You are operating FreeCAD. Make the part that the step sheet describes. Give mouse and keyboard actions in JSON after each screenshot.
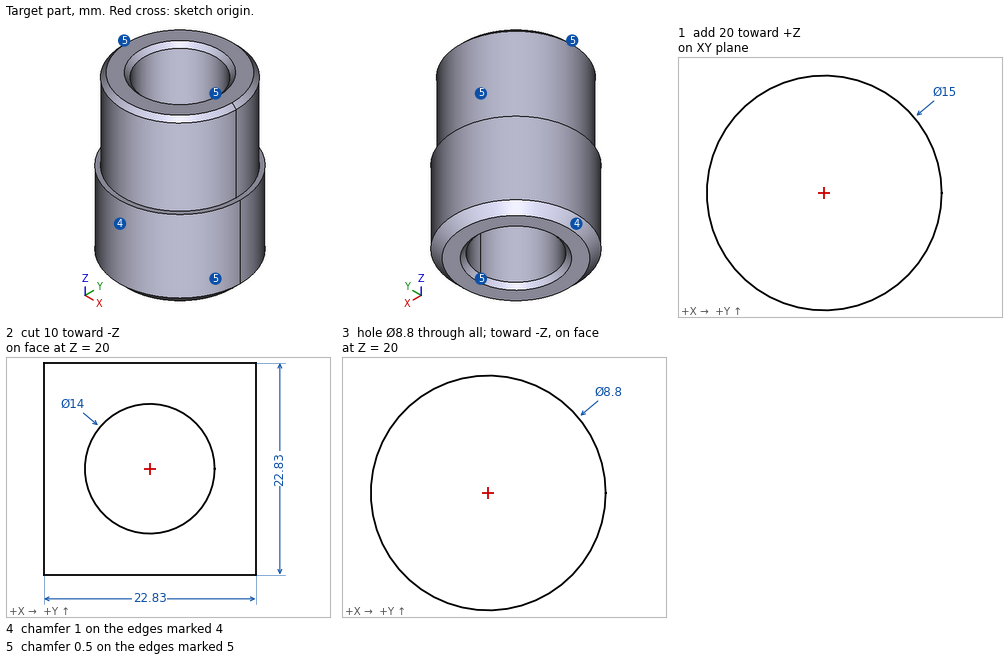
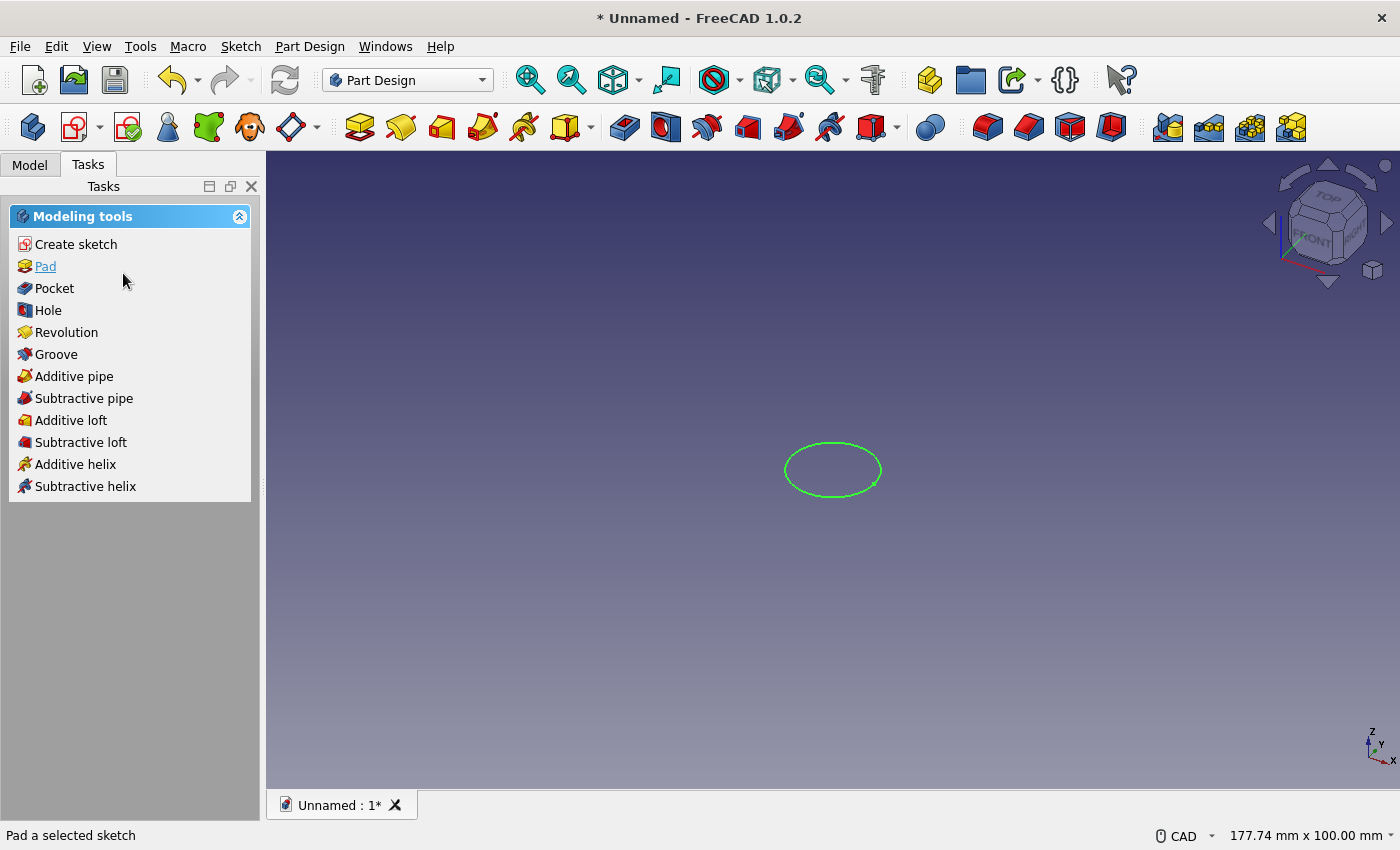
{"action": "left_click", "coordinate": [360, 128]}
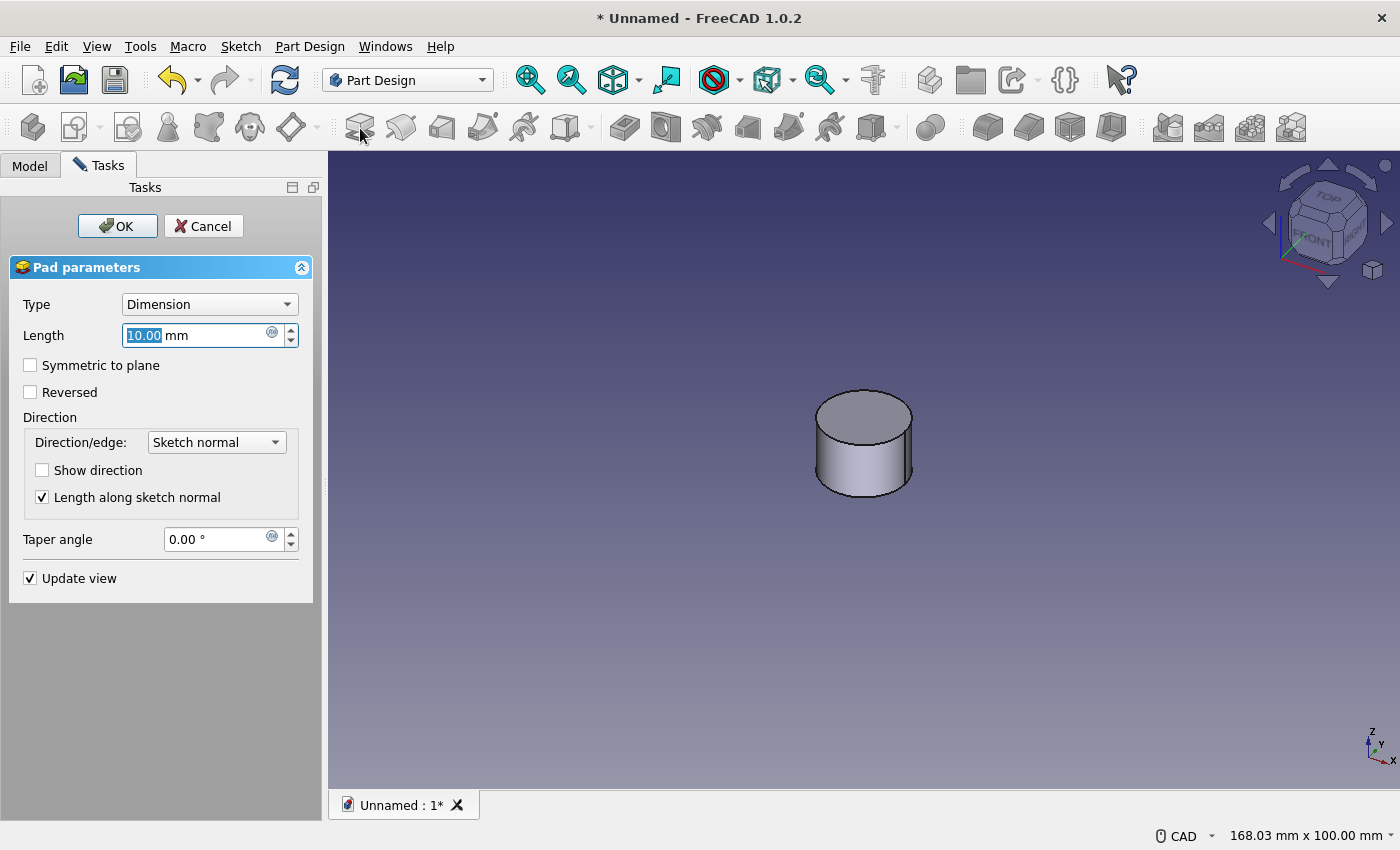
{"action": "type", "text": "20"}
{"action": "key", "text": "Tab"}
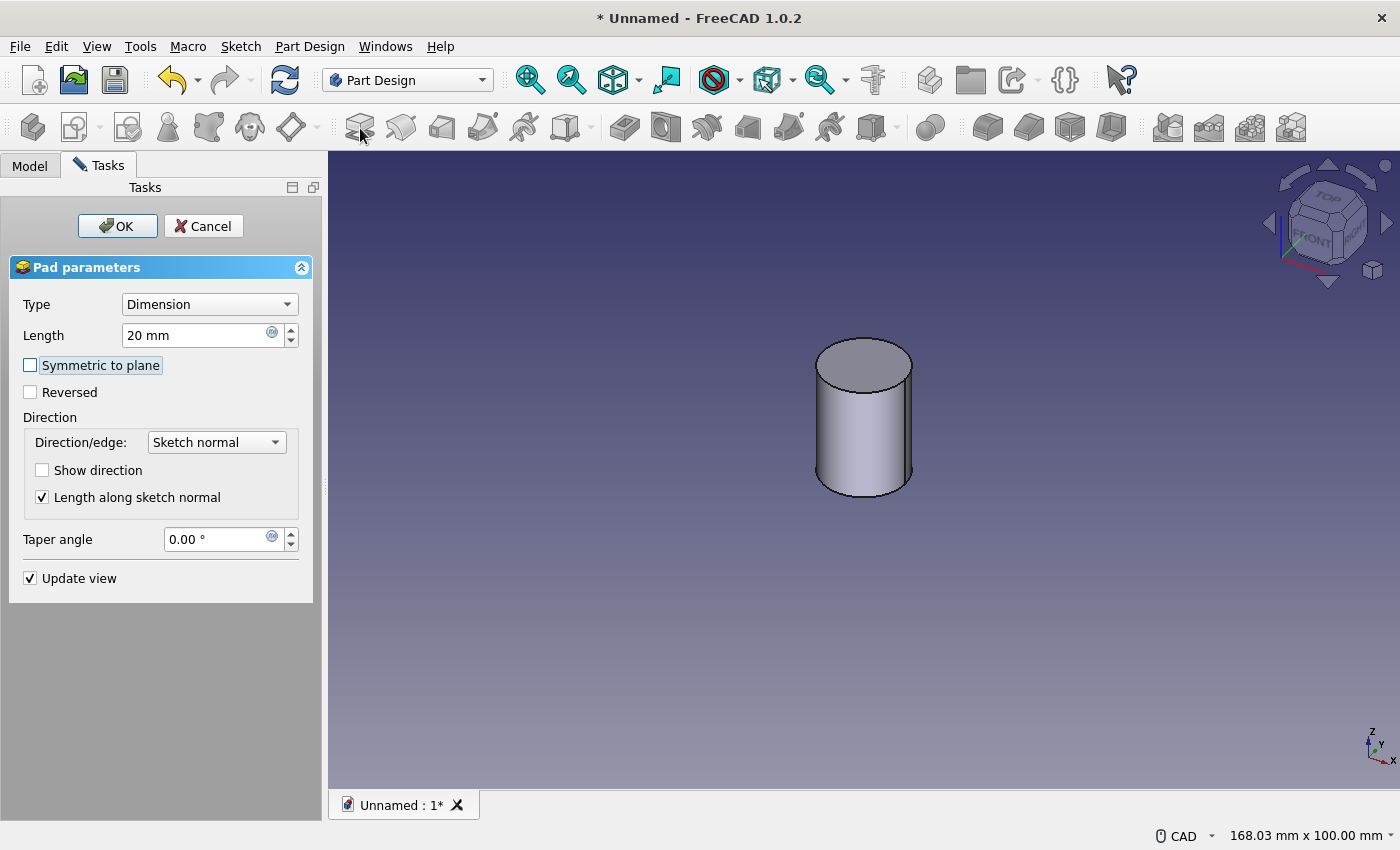
{"action": "left_click", "coordinate": [118, 226]}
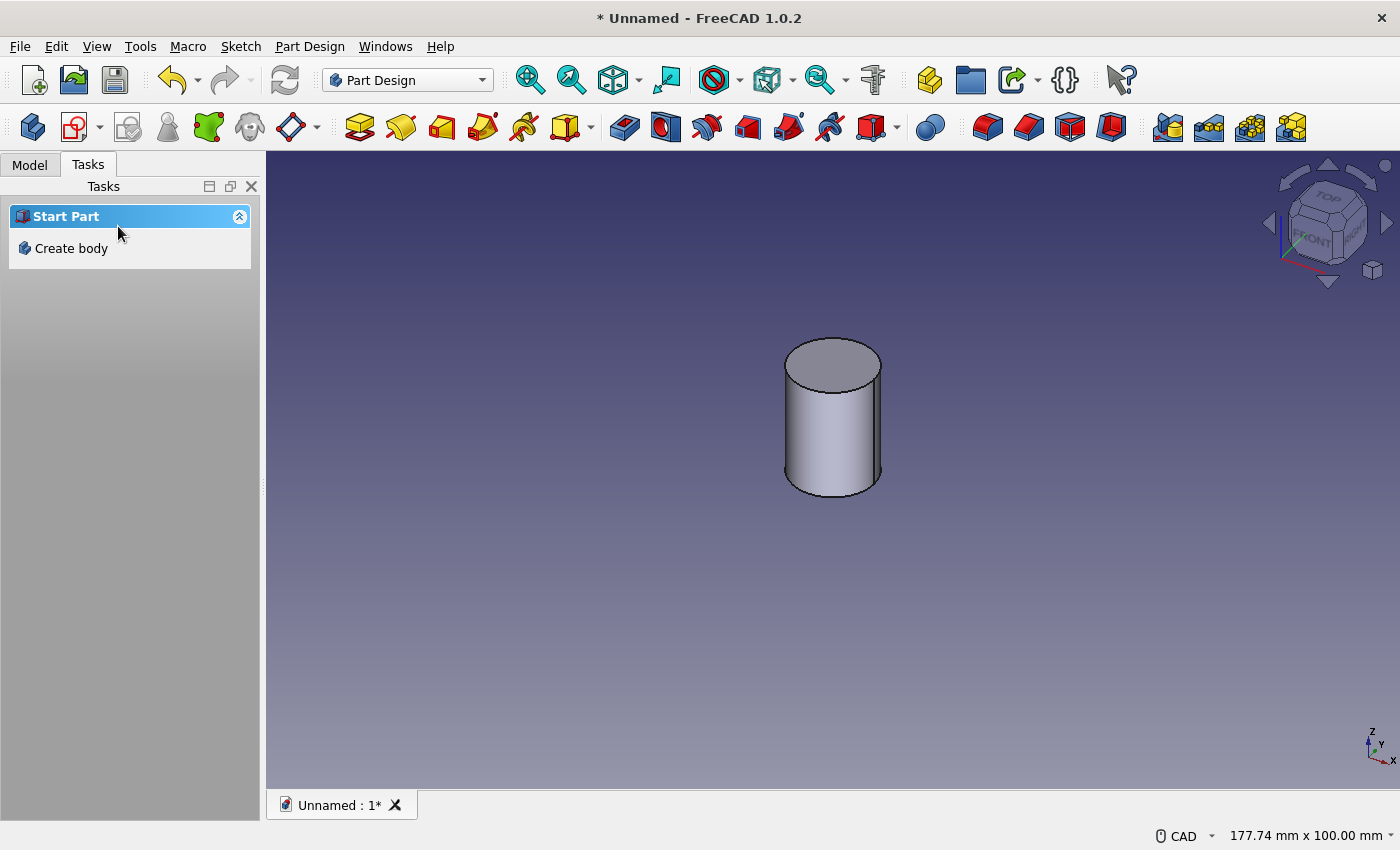
{"action": "left_click", "coordinate": [531, 80]}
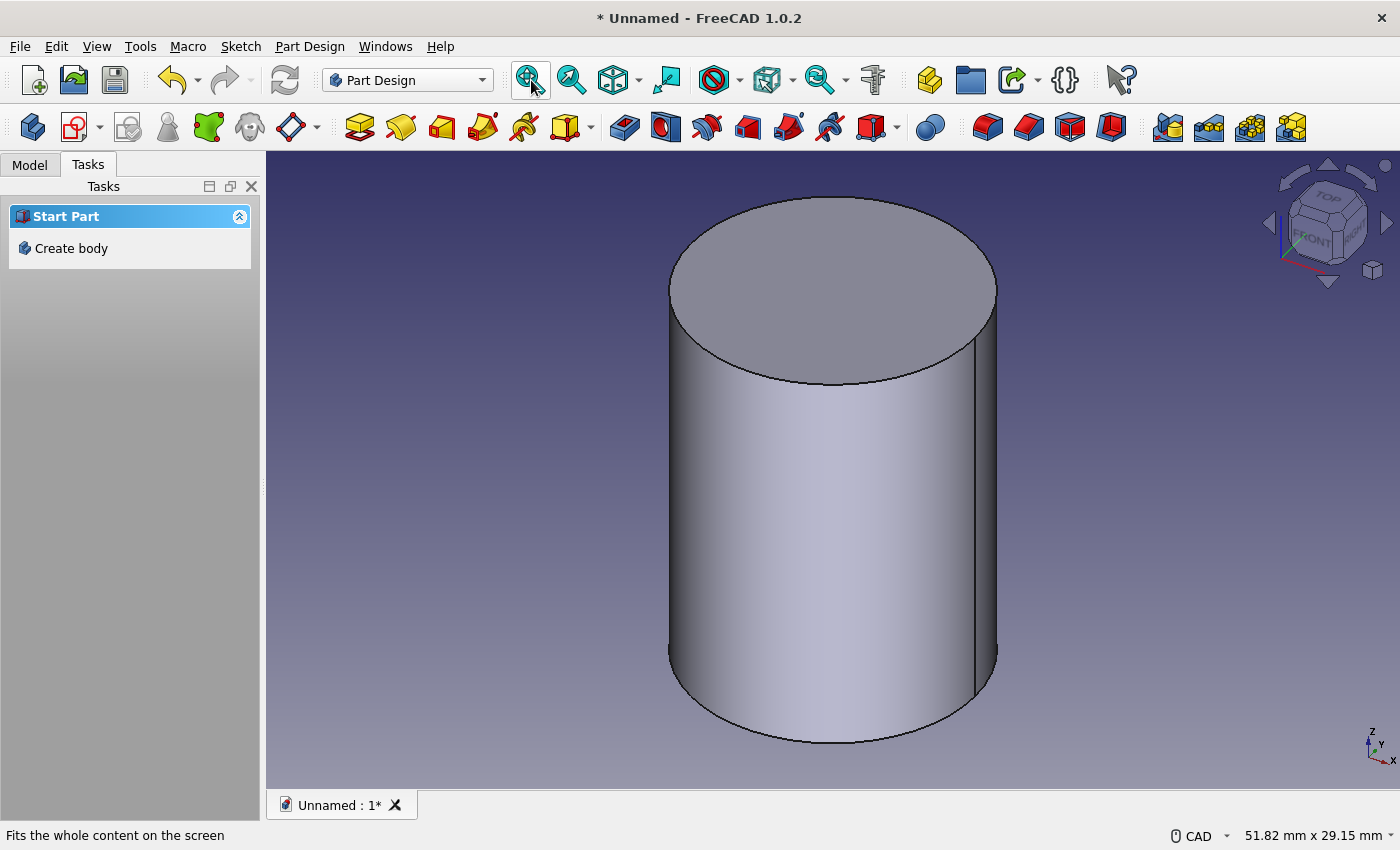
{"action": "left_click", "coordinate": [833, 290]}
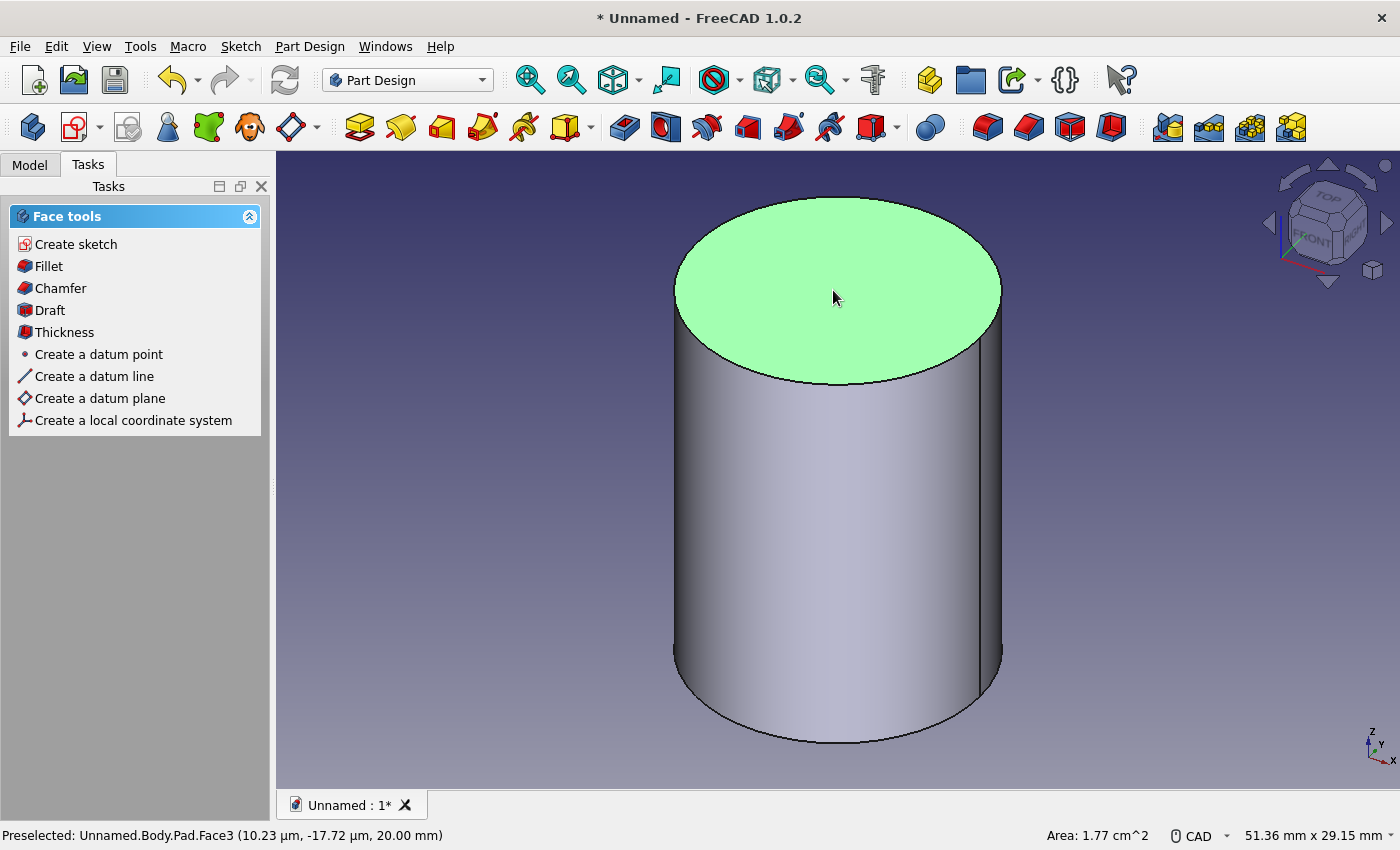
{"action": "left_click", "coordinate": [74, 128]}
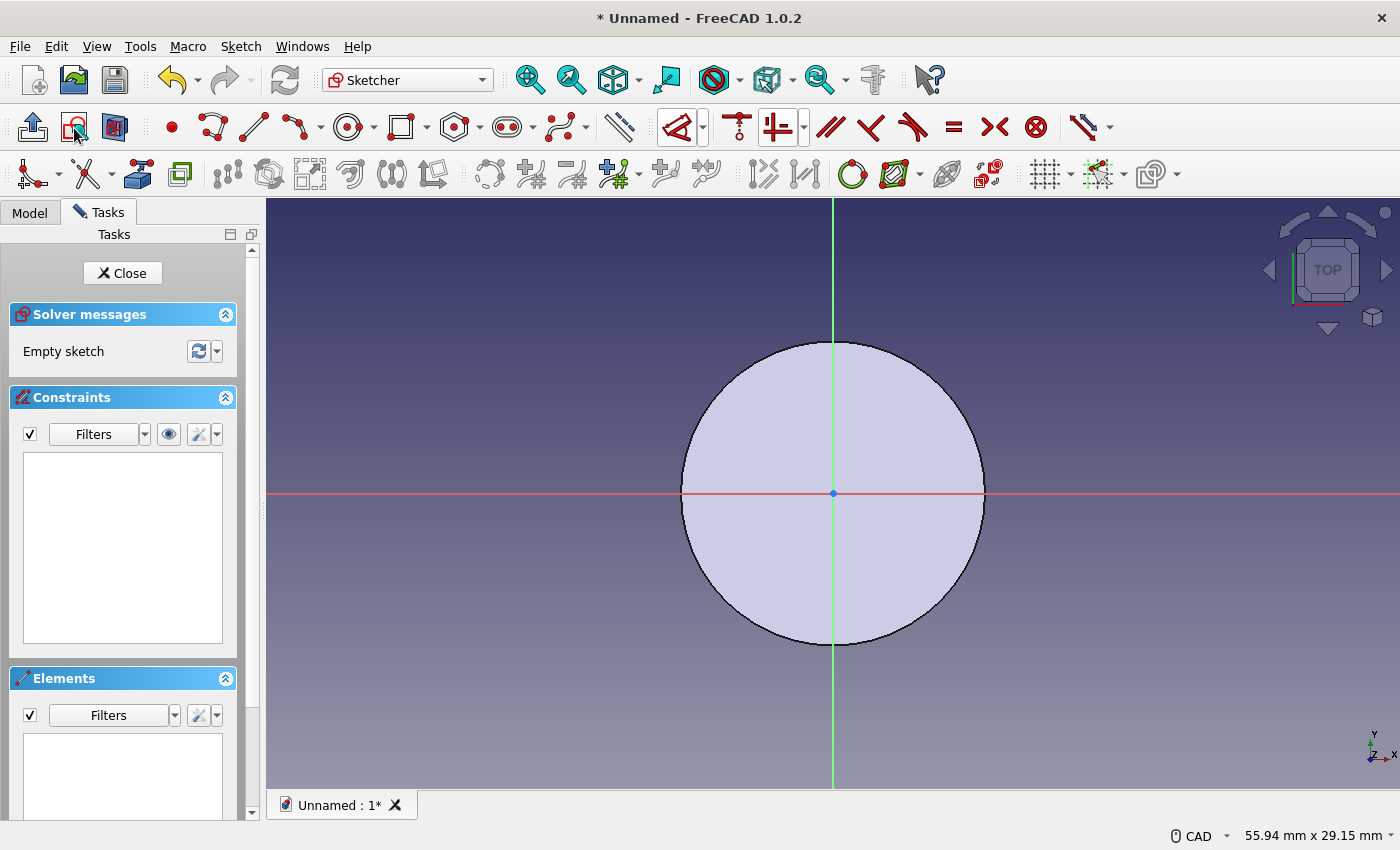
{"action": "key", "text": "g v"}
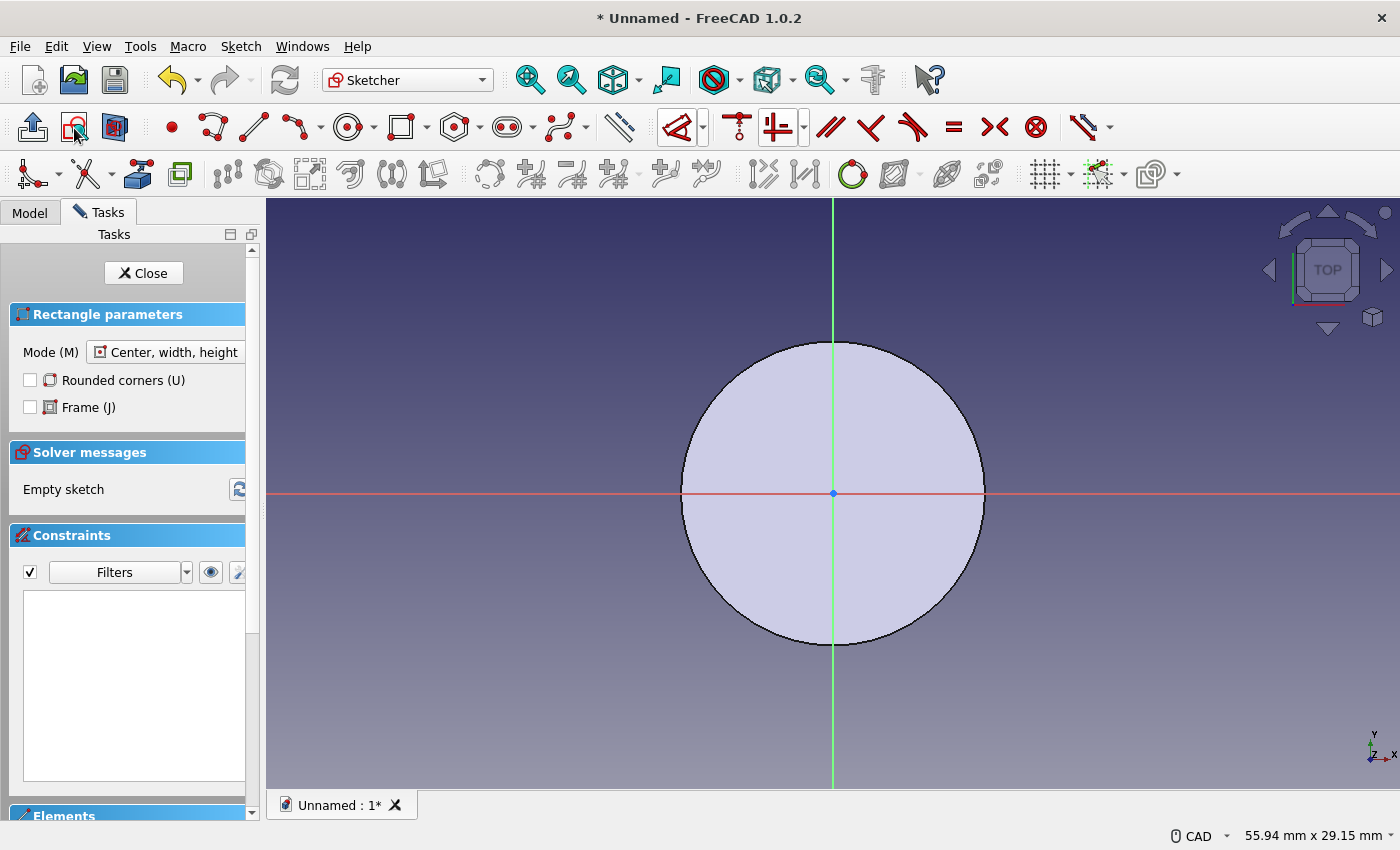
{"action": "left_click", "coordinate": [833, 494]}
{"action": "mouse_move", "coordinate": [1064, 262]}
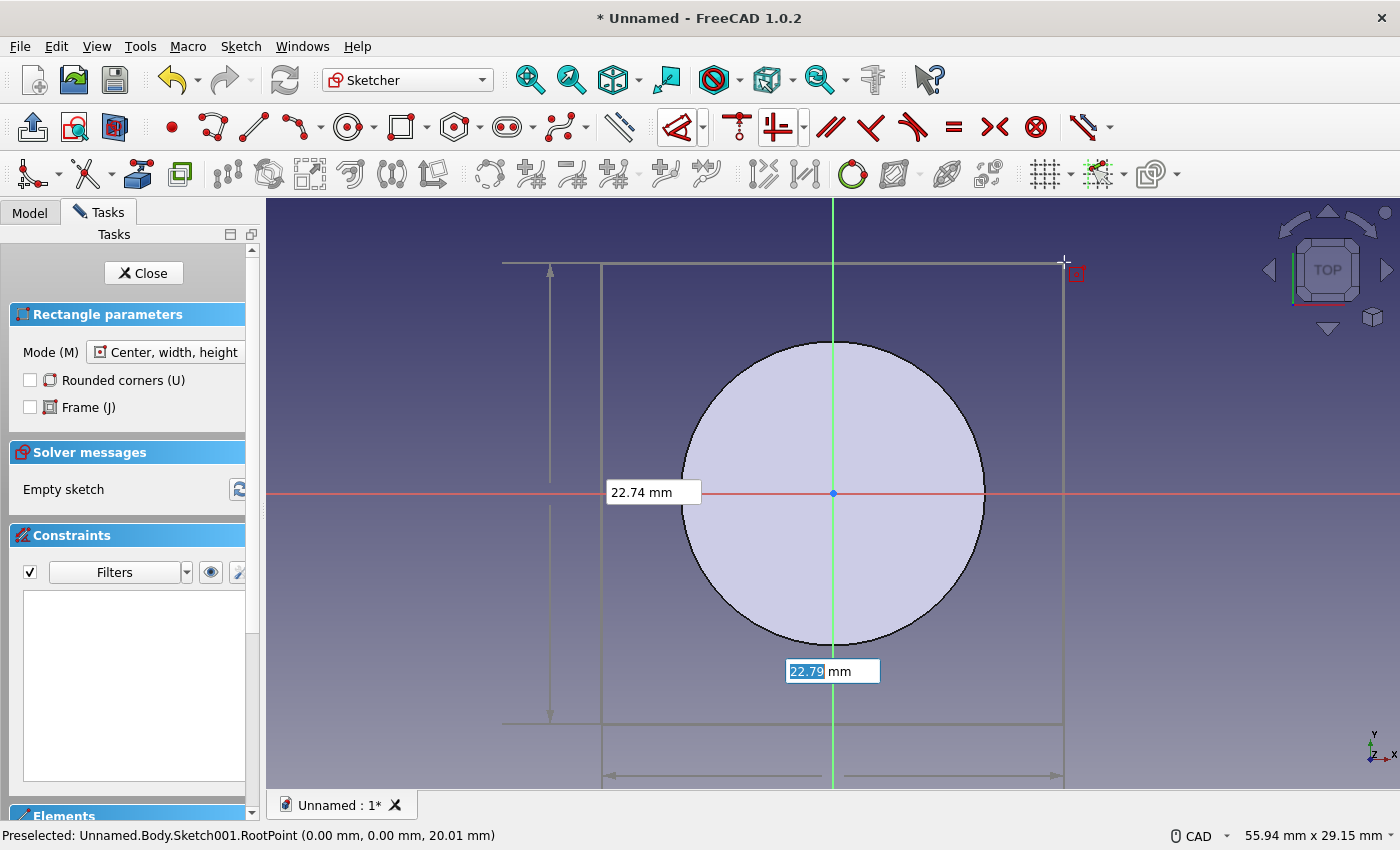
{"action": "type", "text": "22.83"}
{"action": "key", "text": "Tab"}
{"action": "type", "text": "22.83"}
{"action": "key", "text": "Return"}